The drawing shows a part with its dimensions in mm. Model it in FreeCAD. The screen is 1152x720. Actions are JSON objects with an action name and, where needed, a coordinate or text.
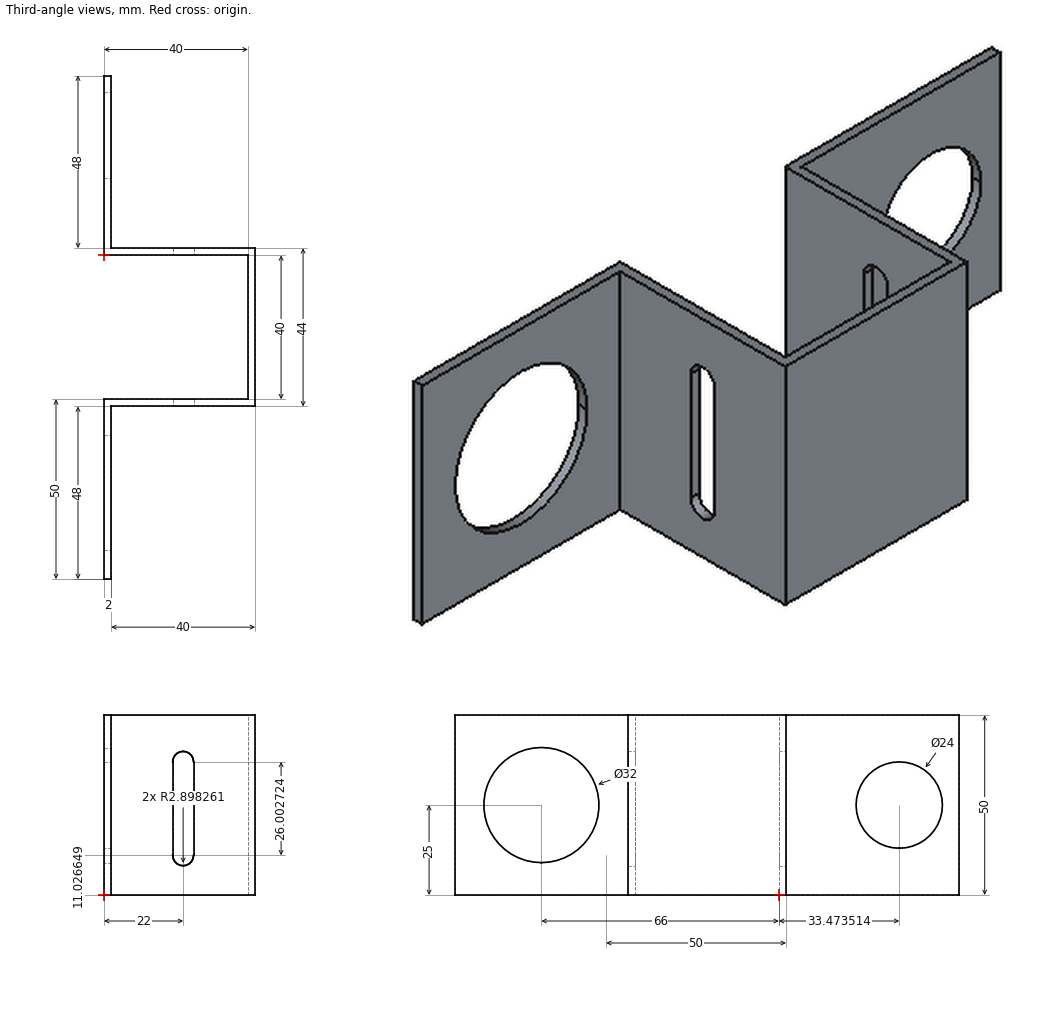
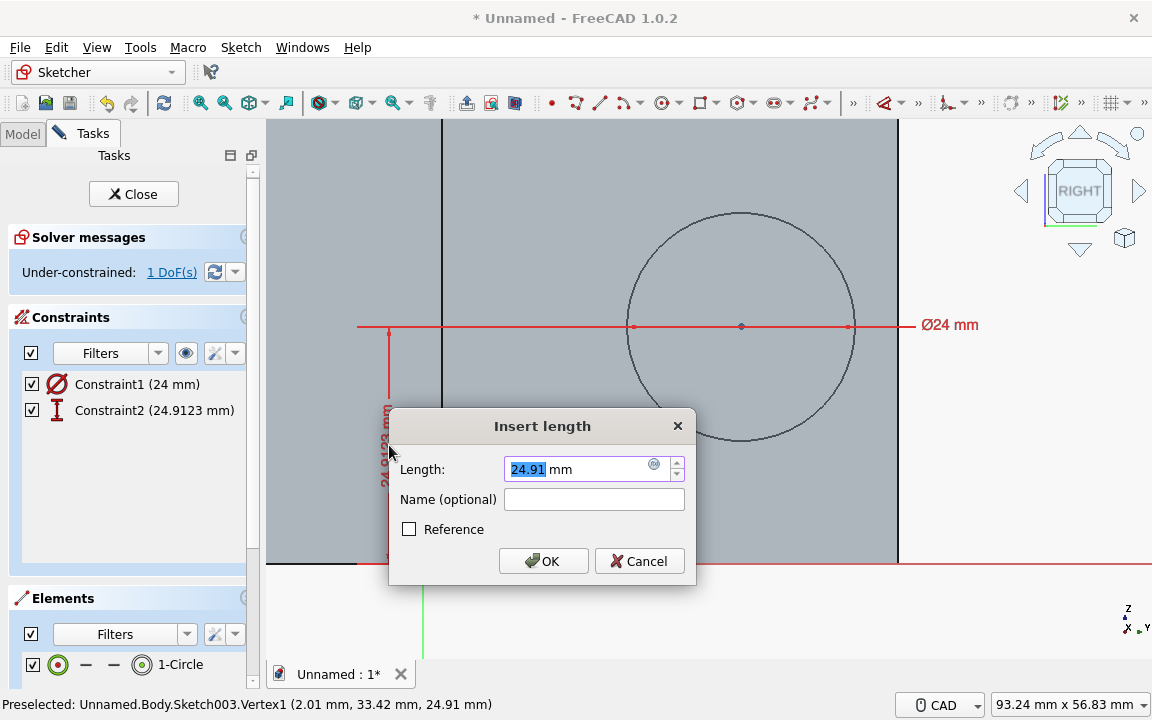
{"action": "type", "text": "25"}
{"action": "key", "text": "Return"}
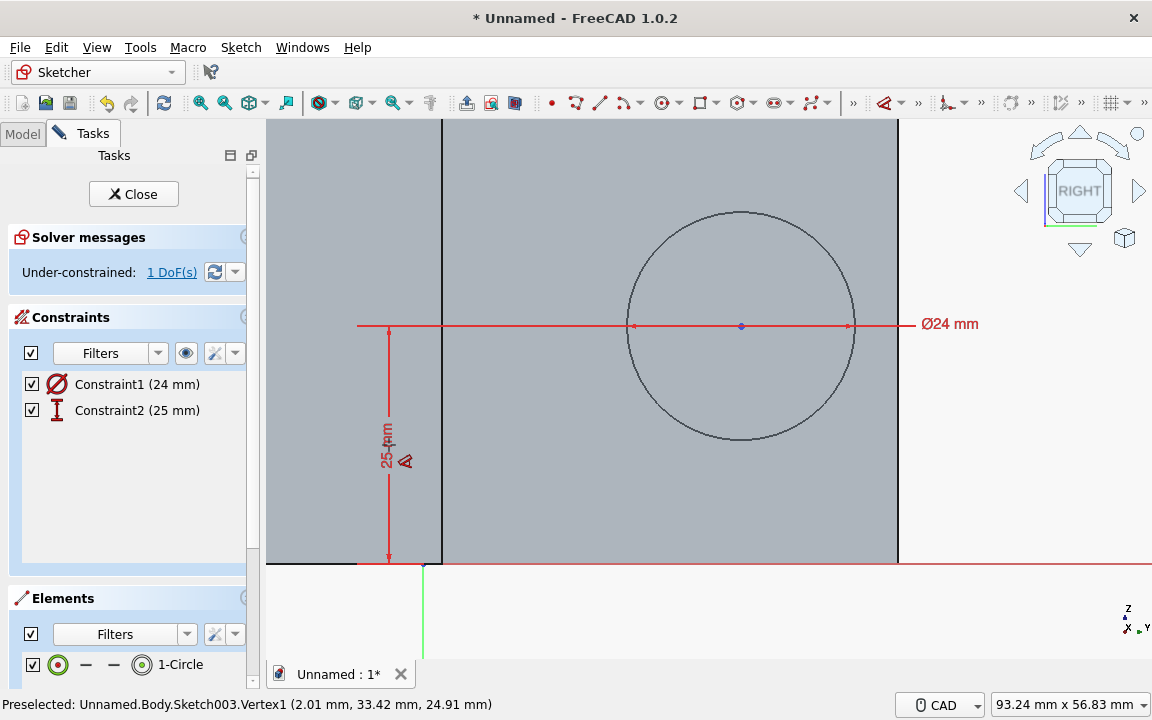
{"action": "left_click", "coordinate": [741, 326]}
{"action": "left_click", "coordinate": [582, 598]}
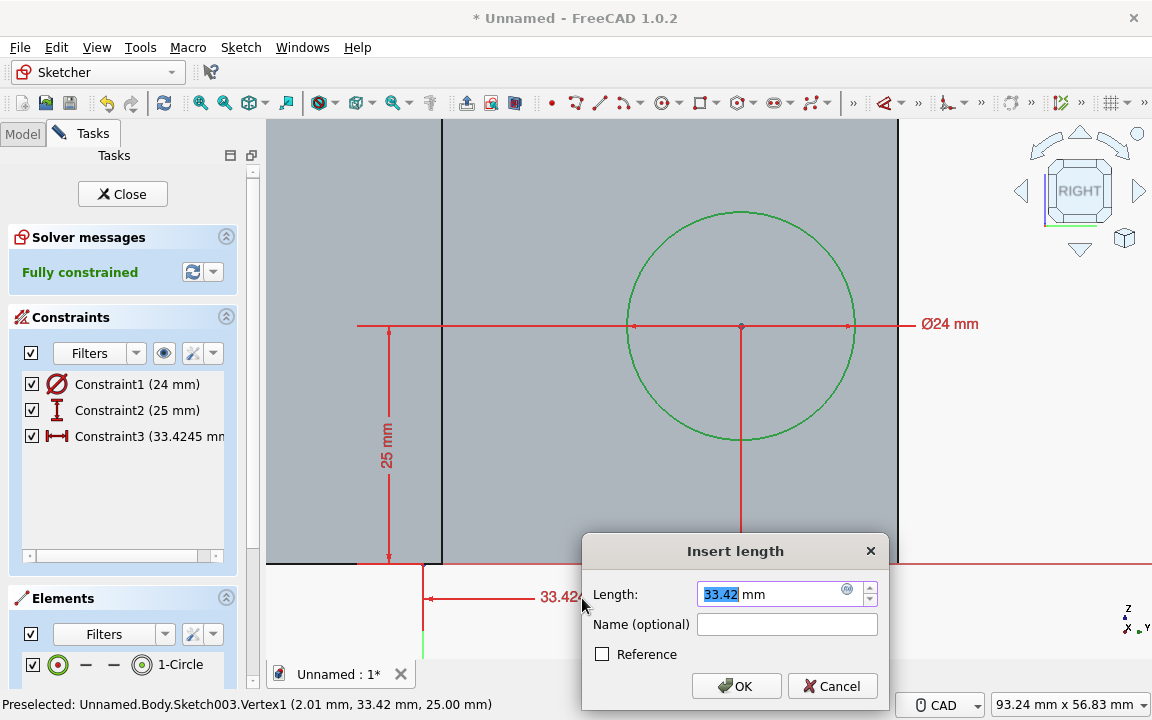
{"action": "type", "text": "33.473514"}
{"action": "key", "text": "Return"}
{"action": "key", "text": "Escape"}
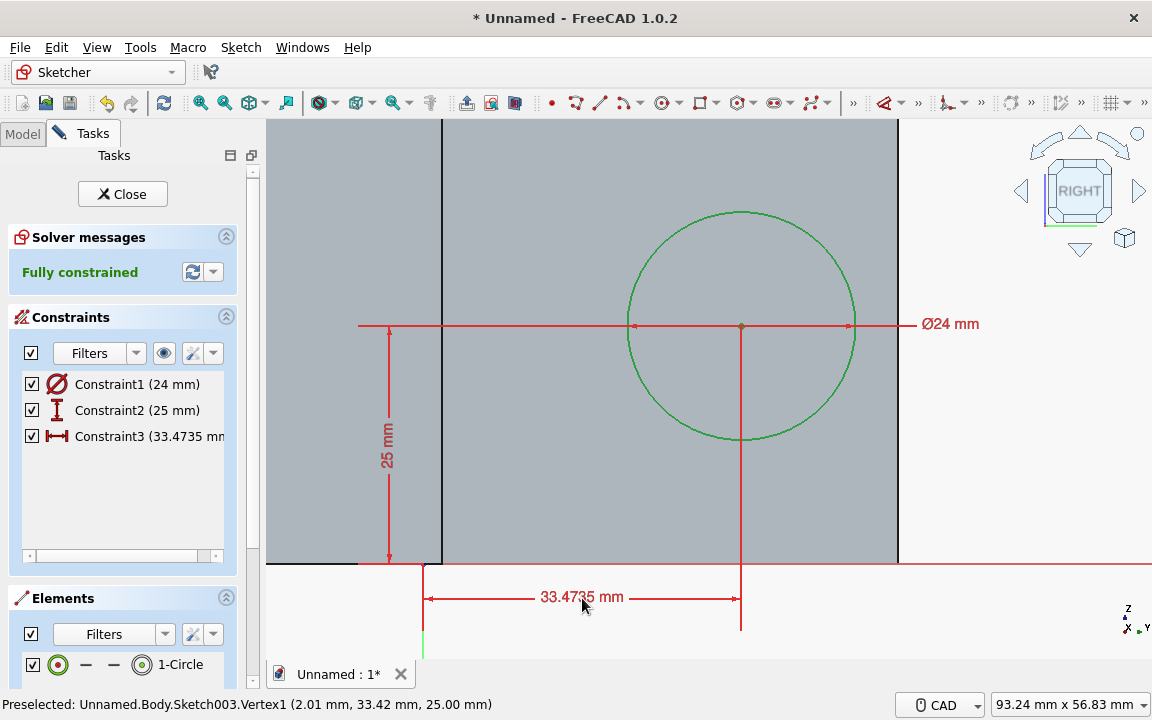
{"action": "left_click", "coordinate": [123, 194]}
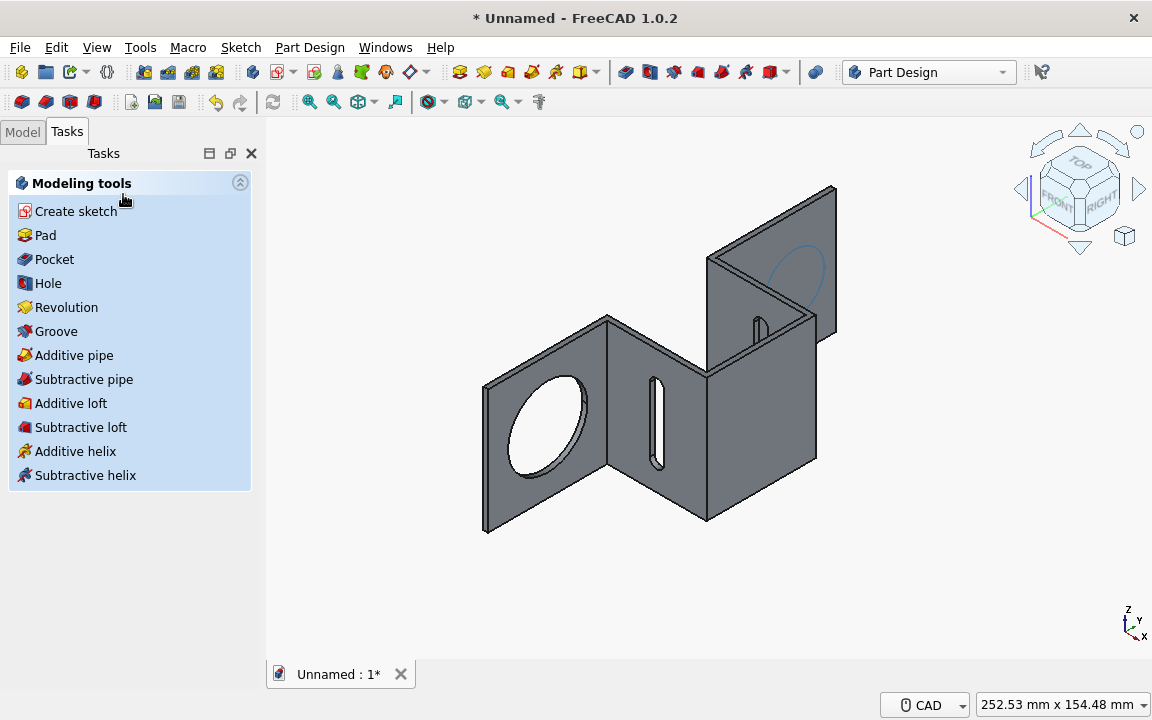
{"action": "left_click", "coordinate": [626, 72]}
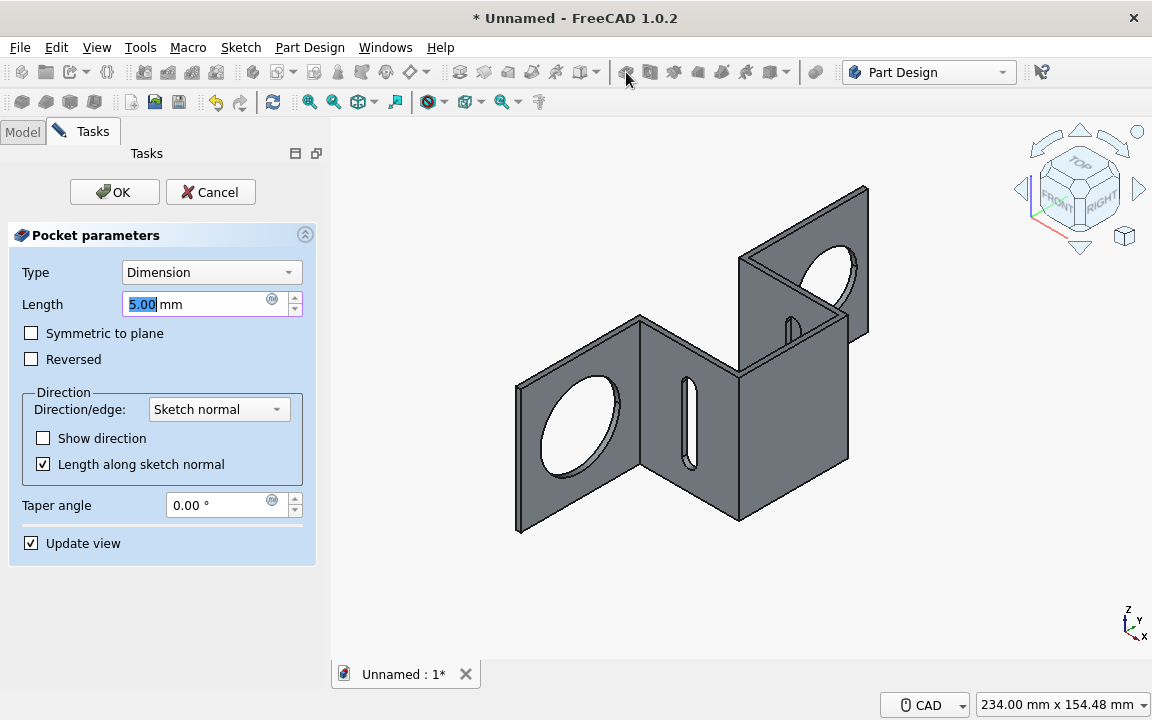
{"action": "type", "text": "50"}
{"action": "key", "text": "Tab"}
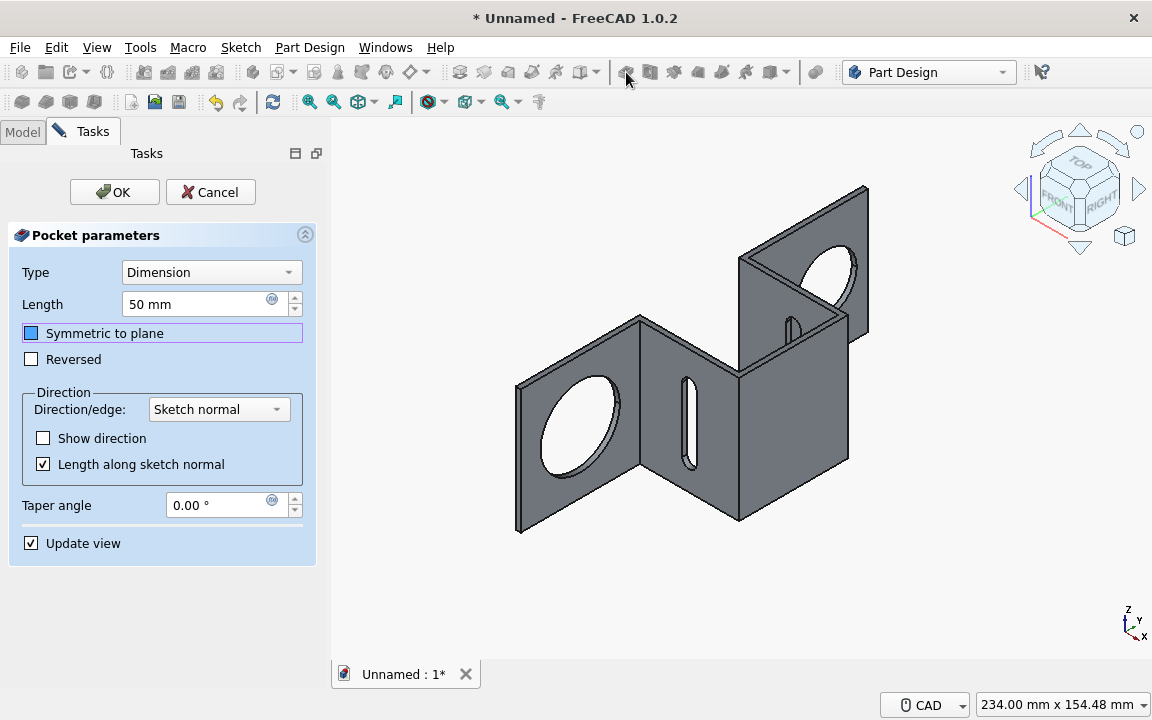
{"action": "left_click", "coordinate": [115, 192]}